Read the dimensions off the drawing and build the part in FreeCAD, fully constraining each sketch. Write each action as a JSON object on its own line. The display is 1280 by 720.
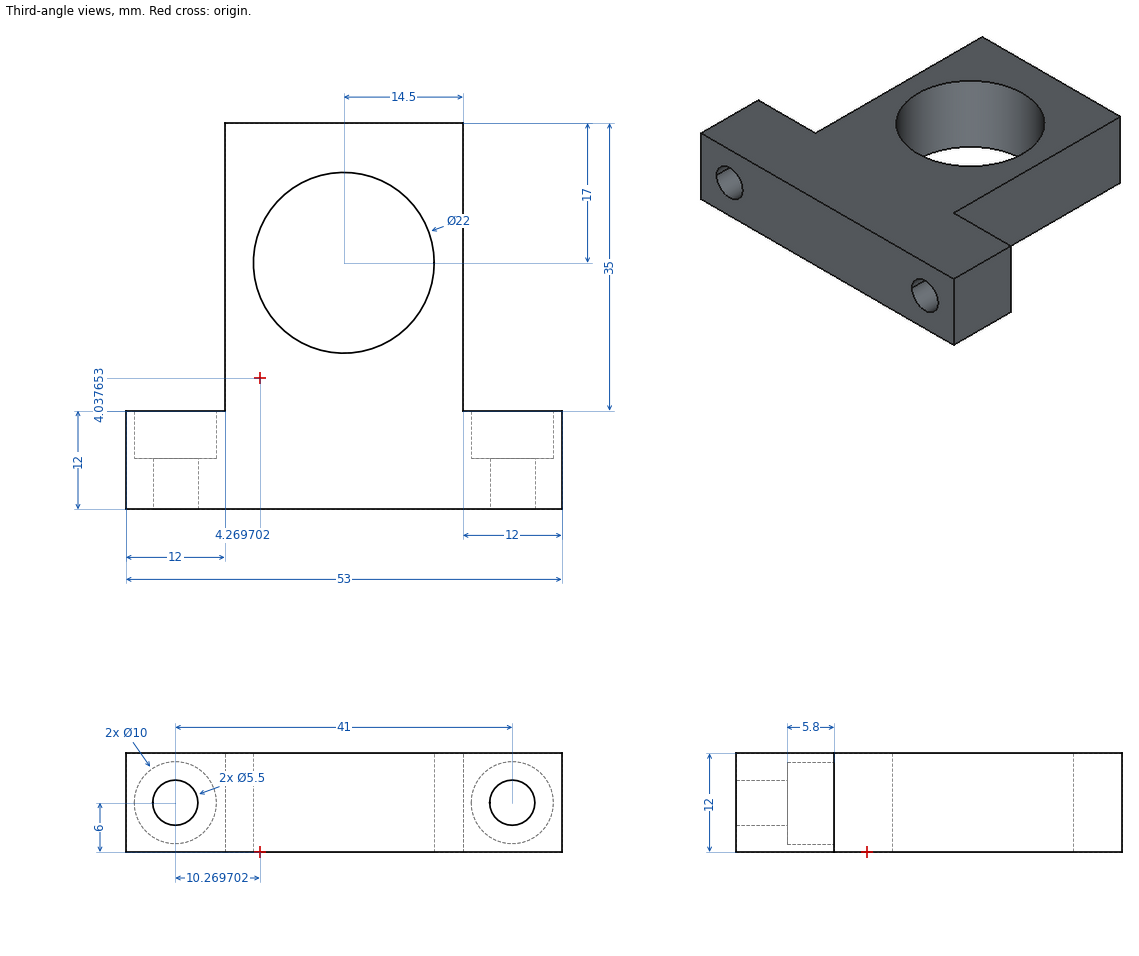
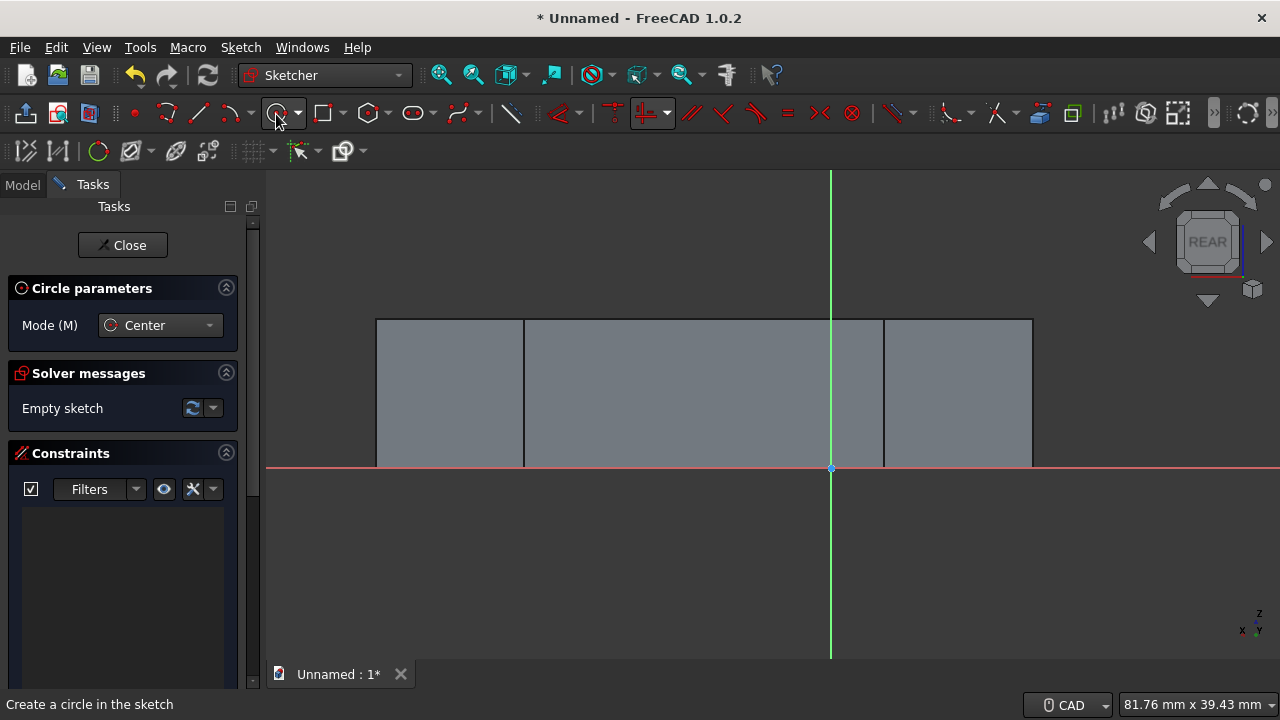
{"action": "left_click", "coordinate": [959, 394]}
{"action": "mouse_move", "coordinate": [983, 370]}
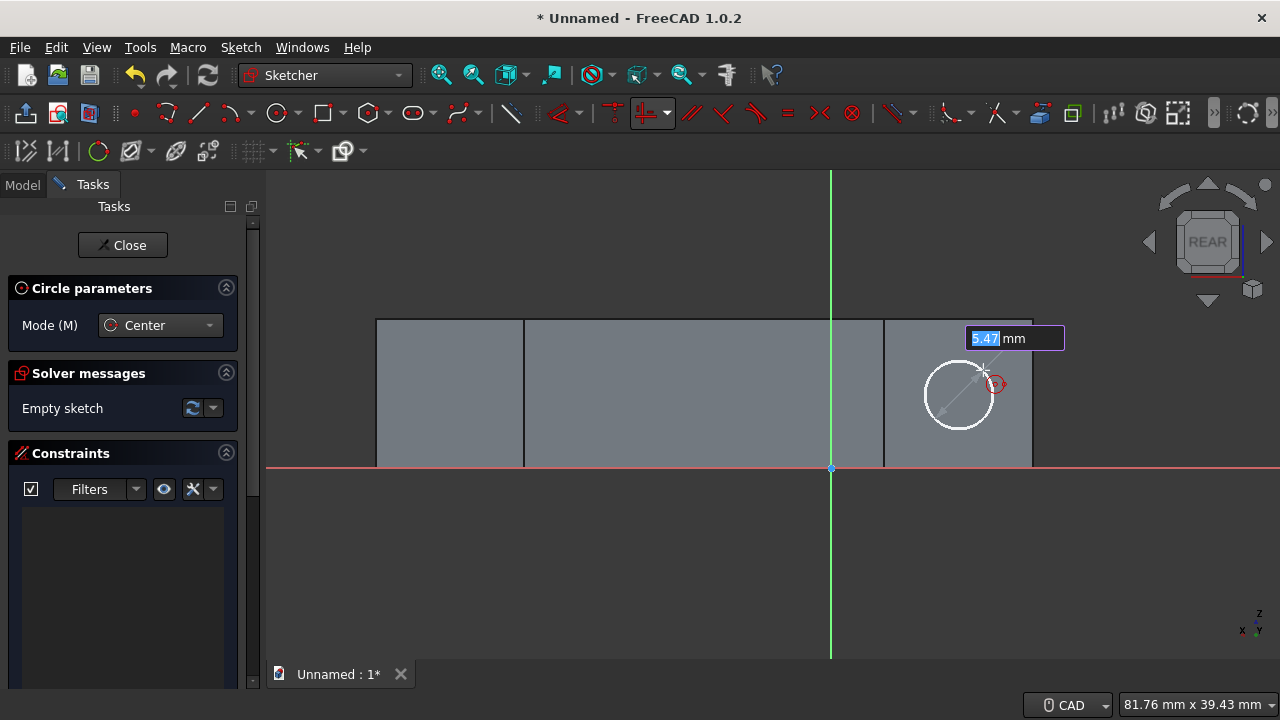
{"action": "type", "text": "5.5"}
{"action": "key", "text": "Return"}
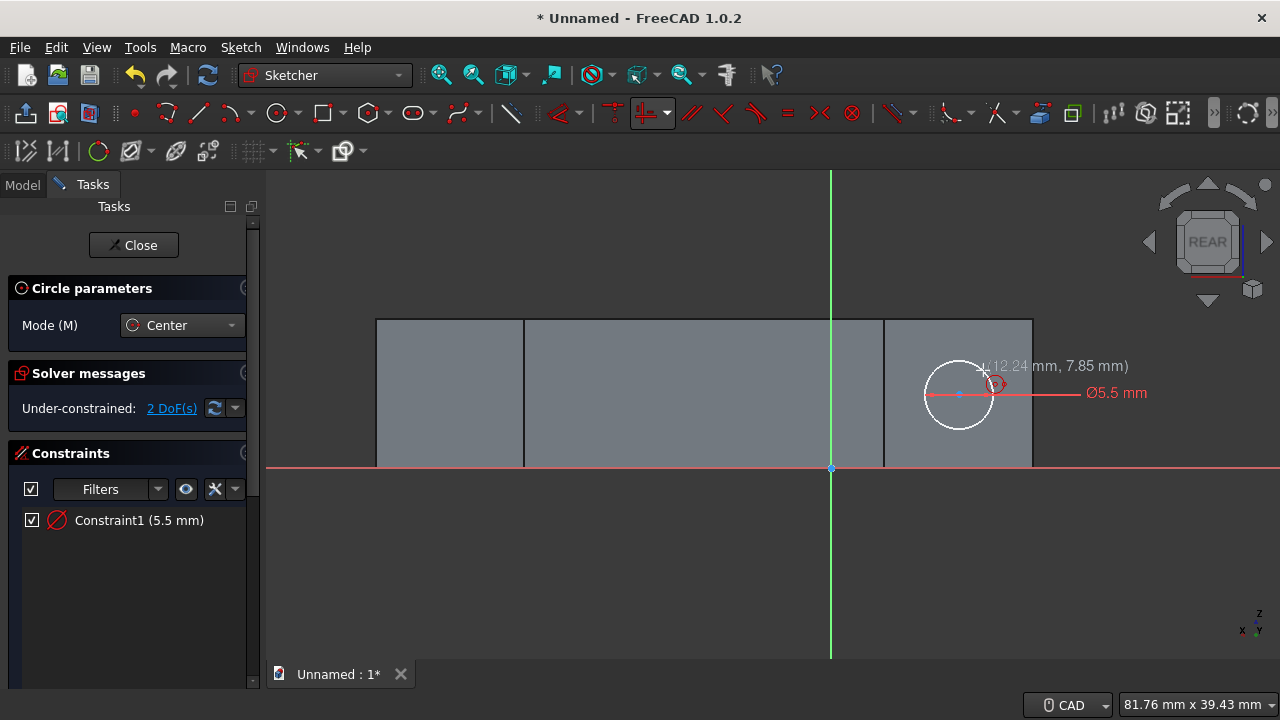
{"action": "left_click", "coordinate": [450, 394]}
{"action": "mouse_move", "coordinate": [474, 370]}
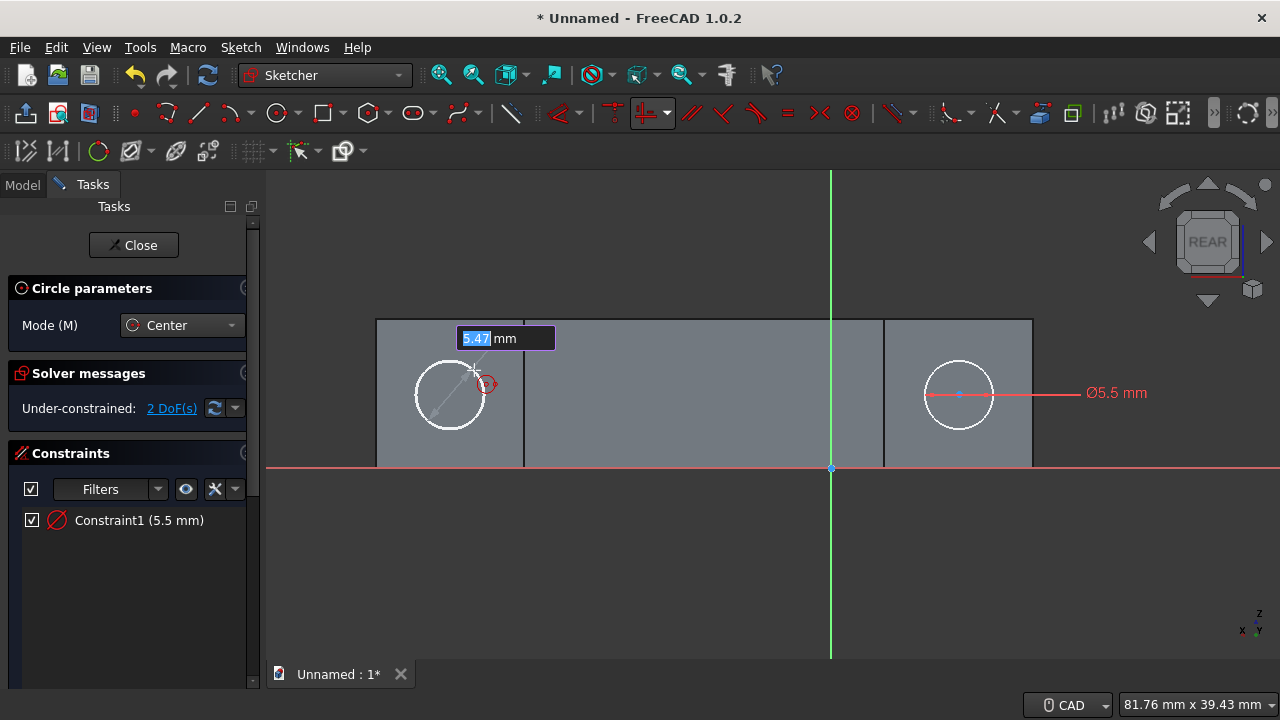
{"action": "type", "text": "5.5"}
{"action": "key", "text": "Return"}
{"action": "key", "text": "Escape"}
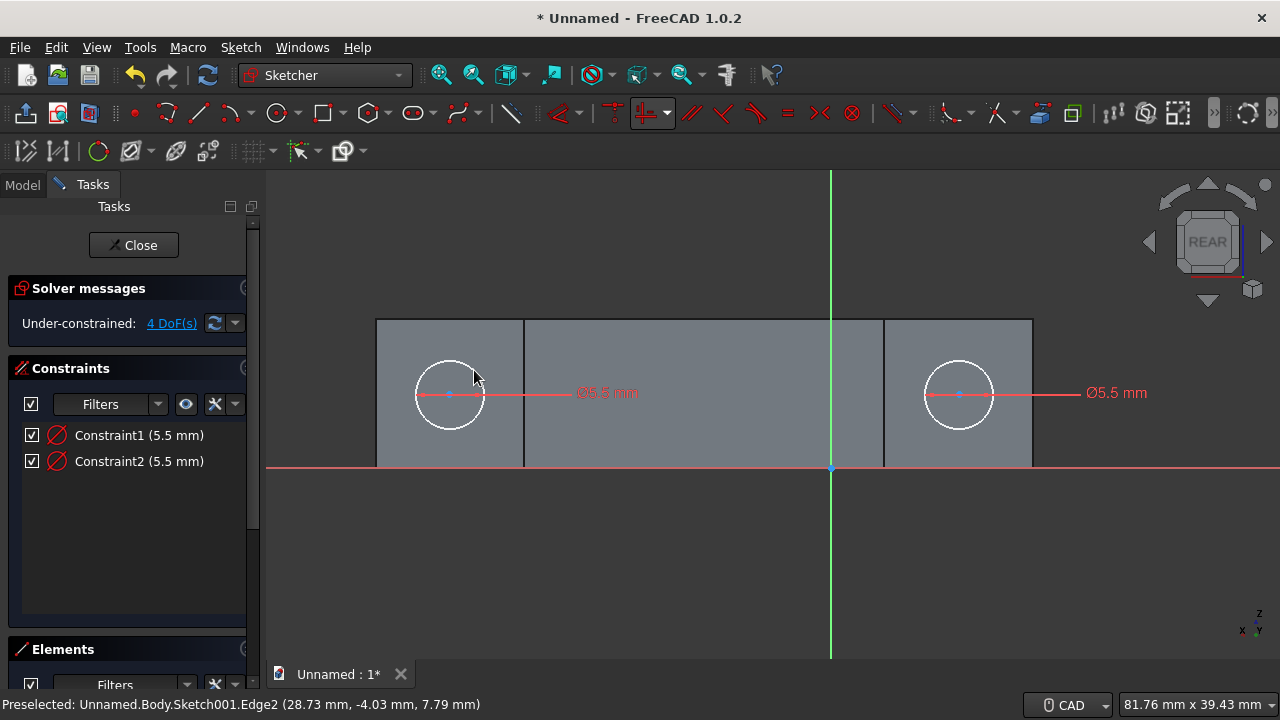
{"action": "left_click", "coordinate": [558, 114]}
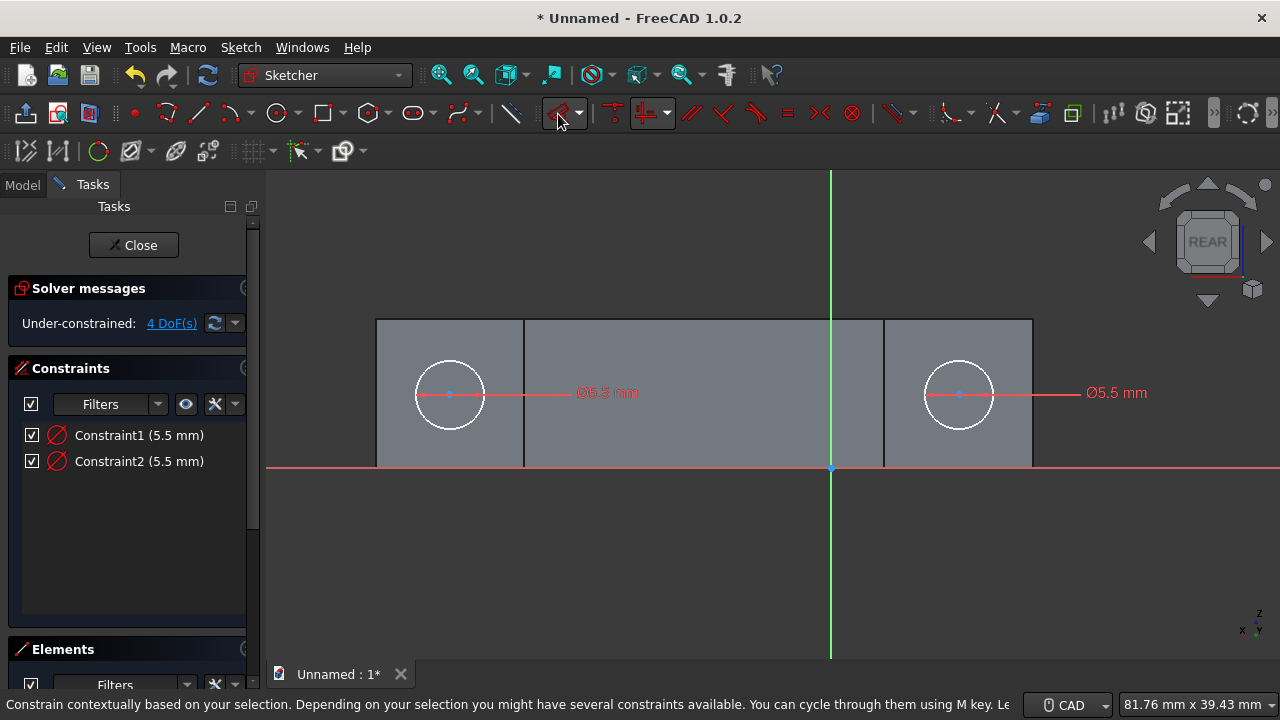
{"action": "left_click", "coordinate": [959, 395]}
{"action": "left_click", "coordinate": [993, 432]}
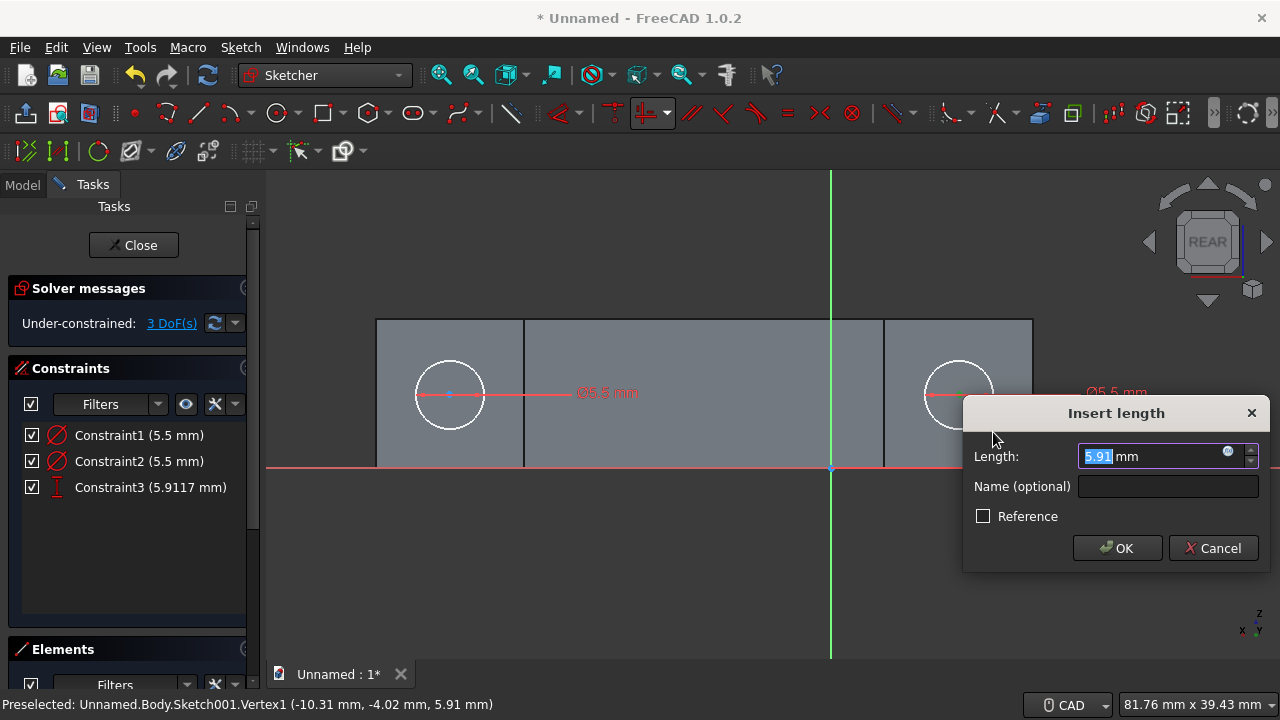
{"action": "type", "text": "6"}
{"action": "key", "text": "Return"}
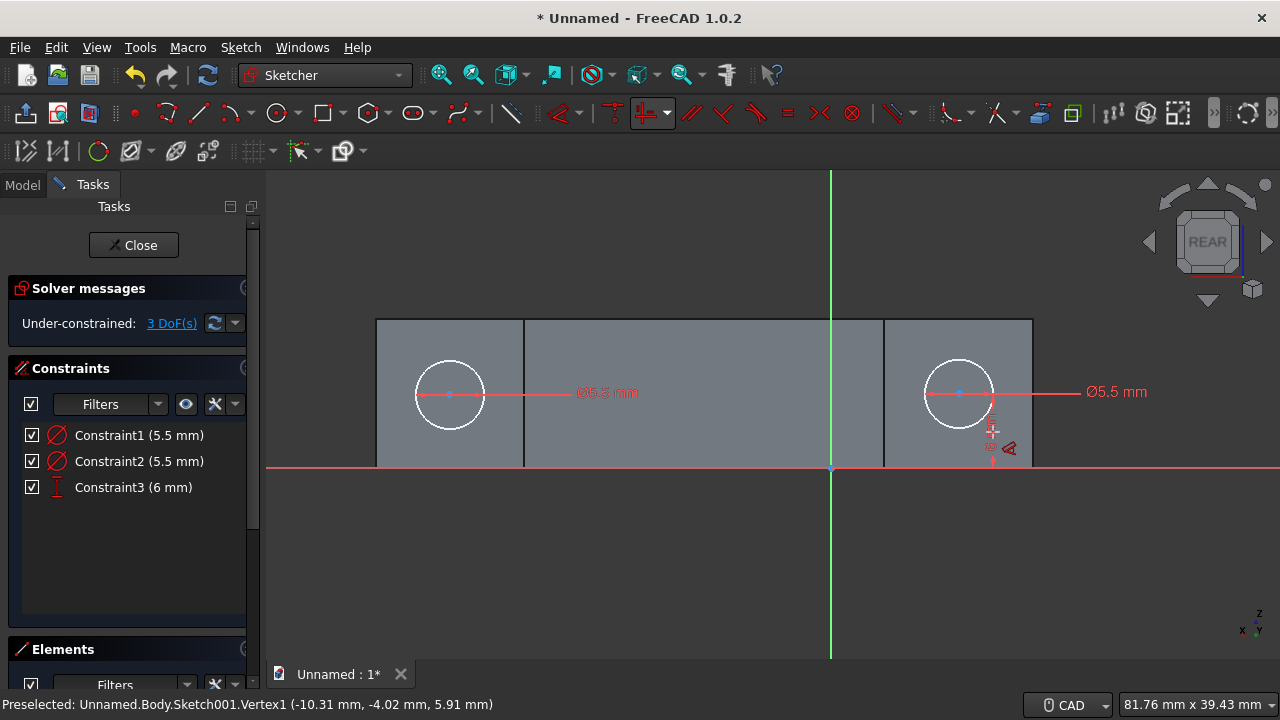
{"action": "left_click", "coordinate": [450, 395]}
{"action": "left_click", "coordinate": [416, 432]}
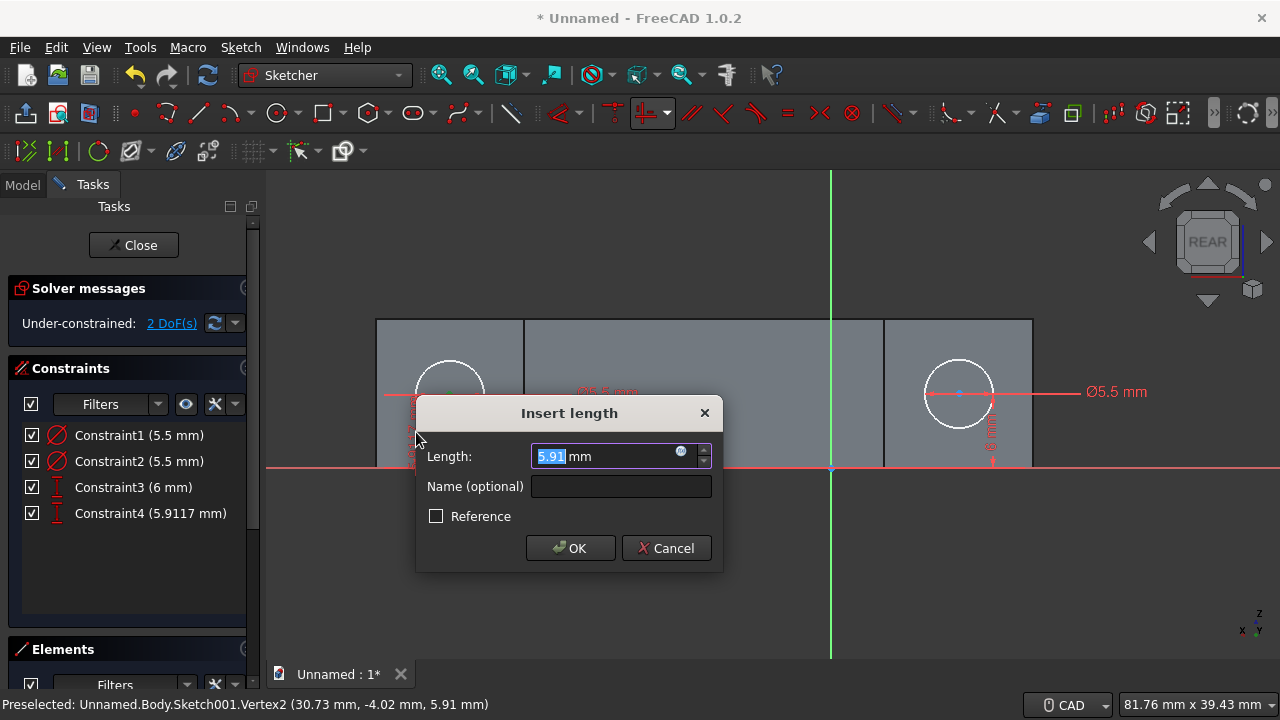
{"action": "type", "text": "6"}
{"action": "key", "text": "Return"}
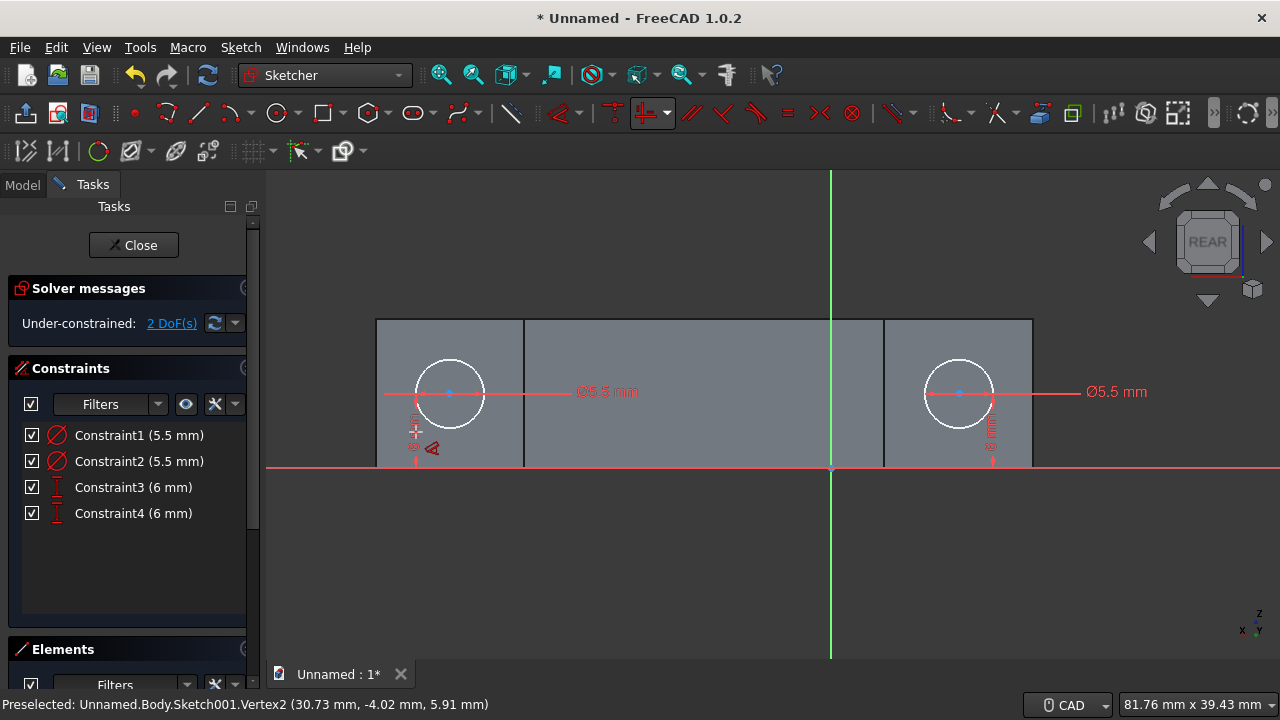
{"action": "left_click", "coordinate": [959, 394]}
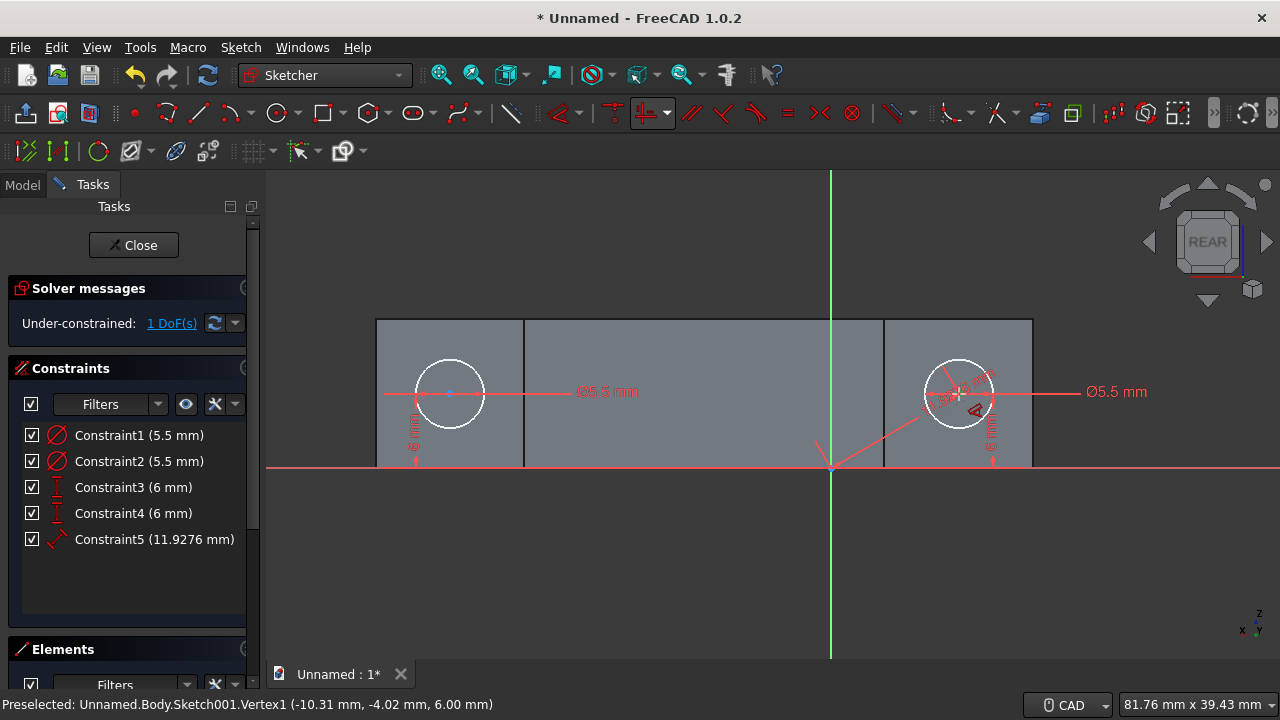
{"action": "left_click", "coordinate": [450, 394]}
{"action": "left_click", "coordinate": [704, 360]}